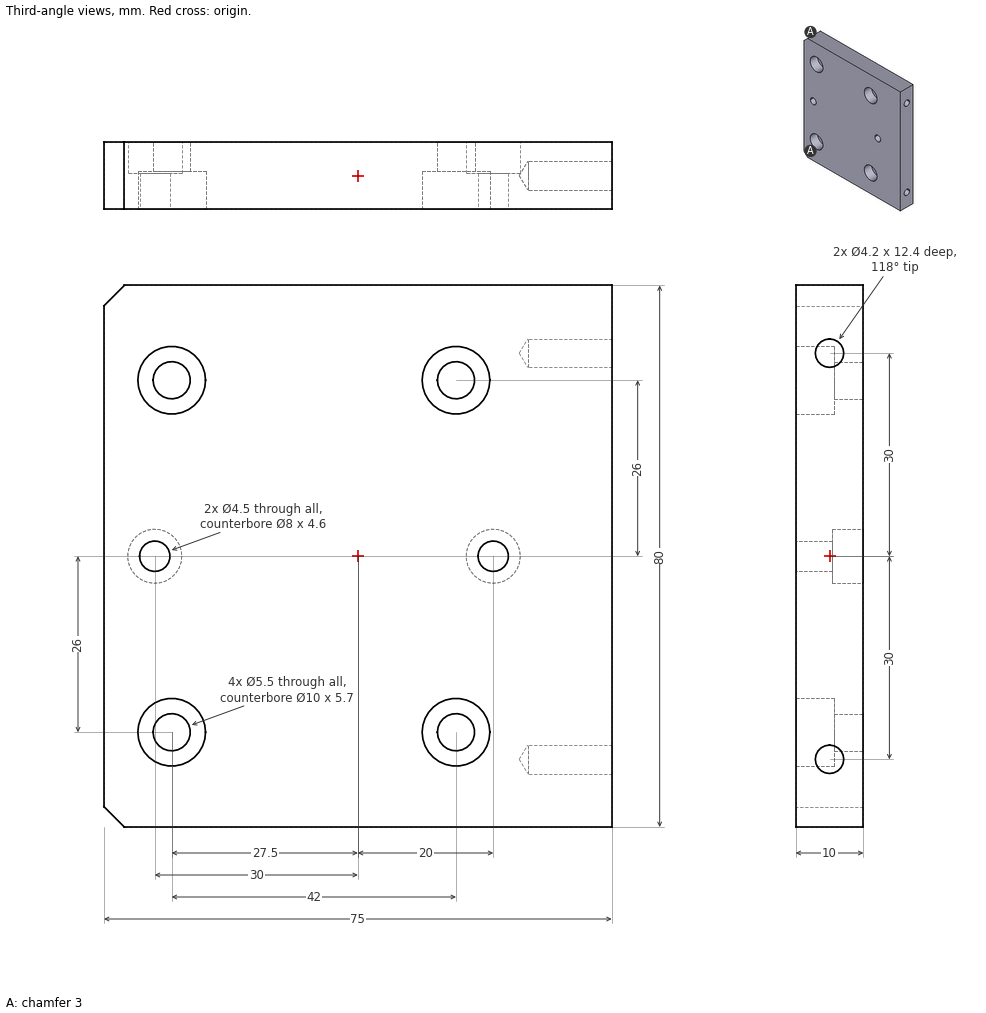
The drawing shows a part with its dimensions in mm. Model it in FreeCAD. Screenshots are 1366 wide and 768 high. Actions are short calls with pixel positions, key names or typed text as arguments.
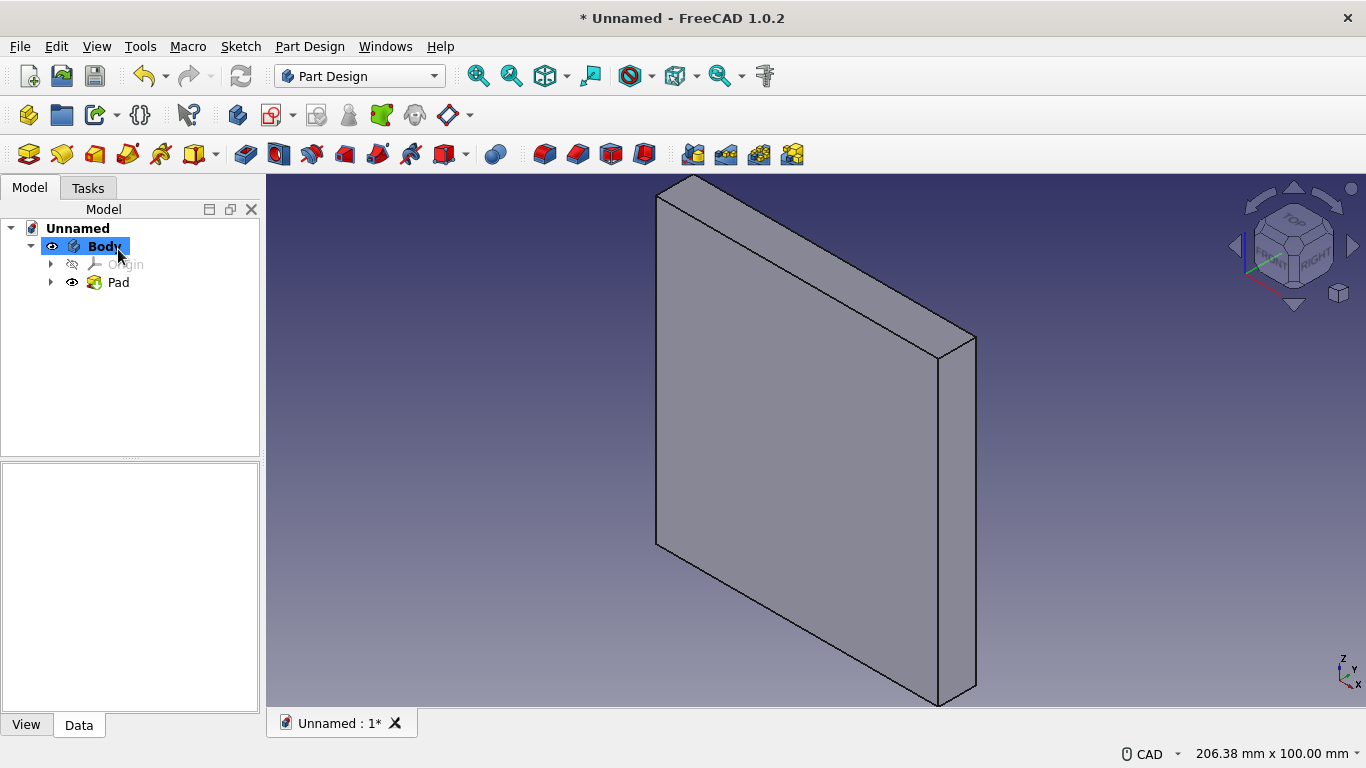
click(479, 76)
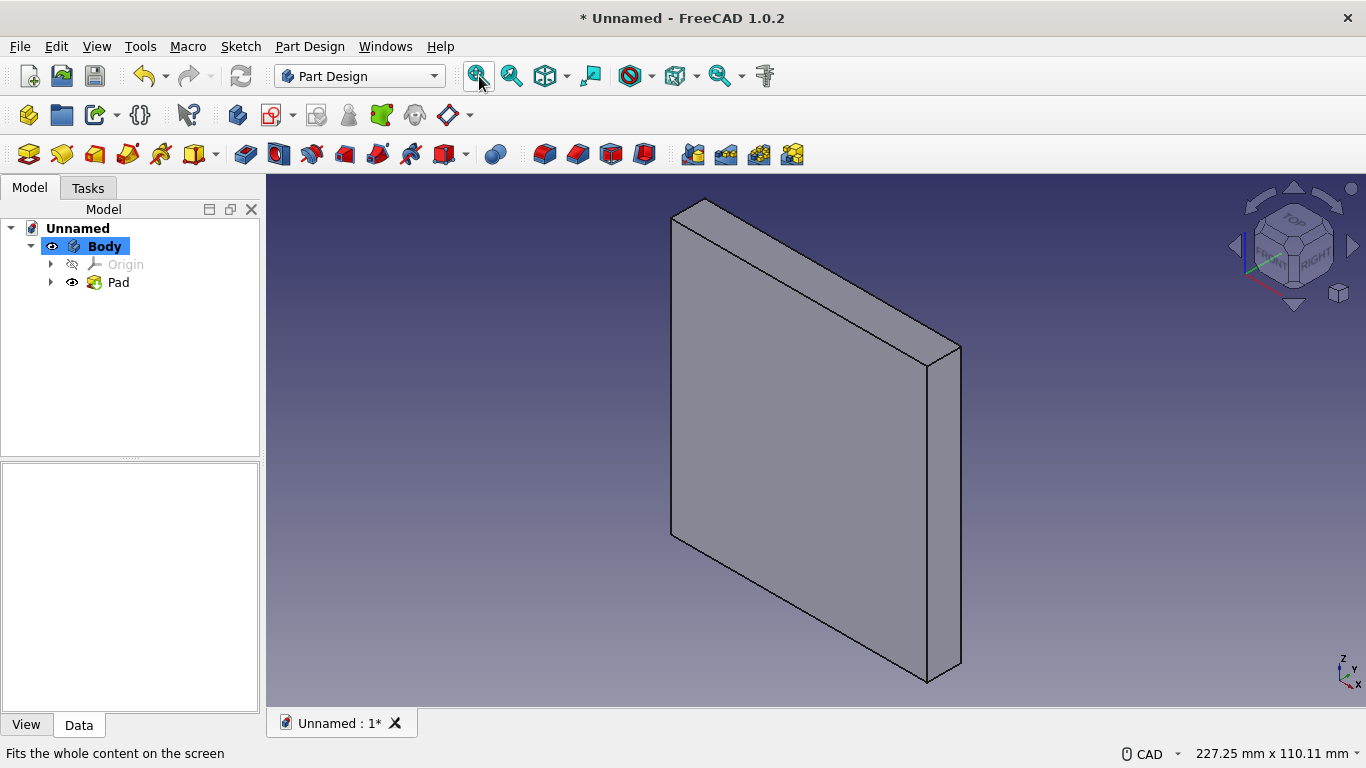
key(2)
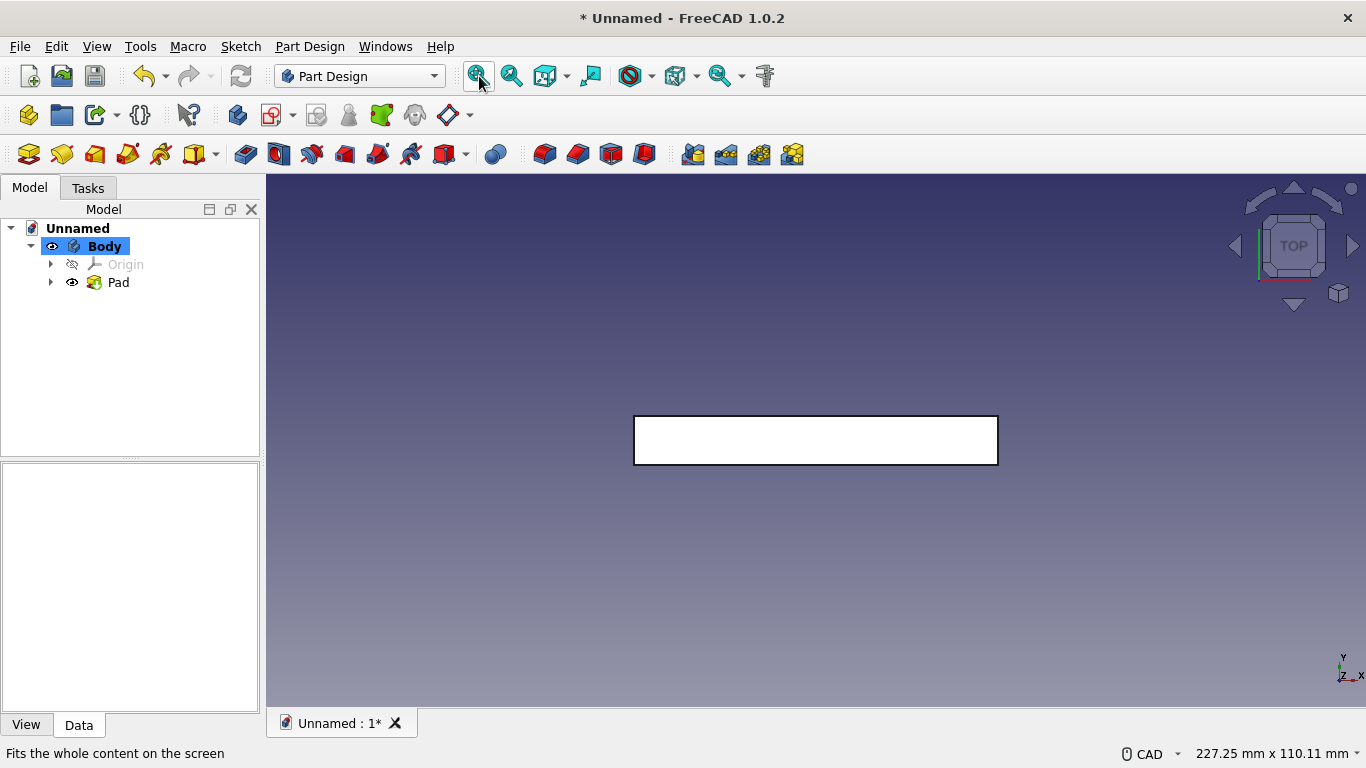
click(479, 76)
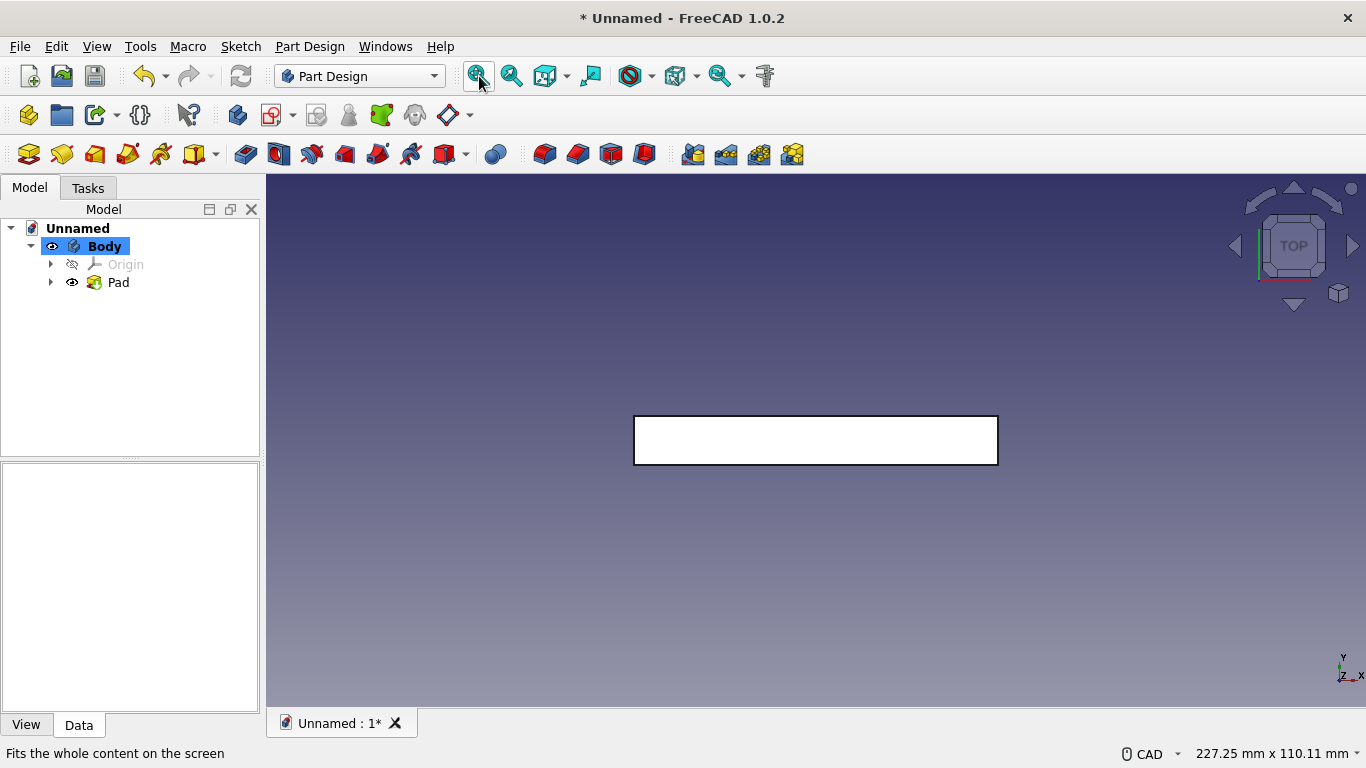
click(634, 439)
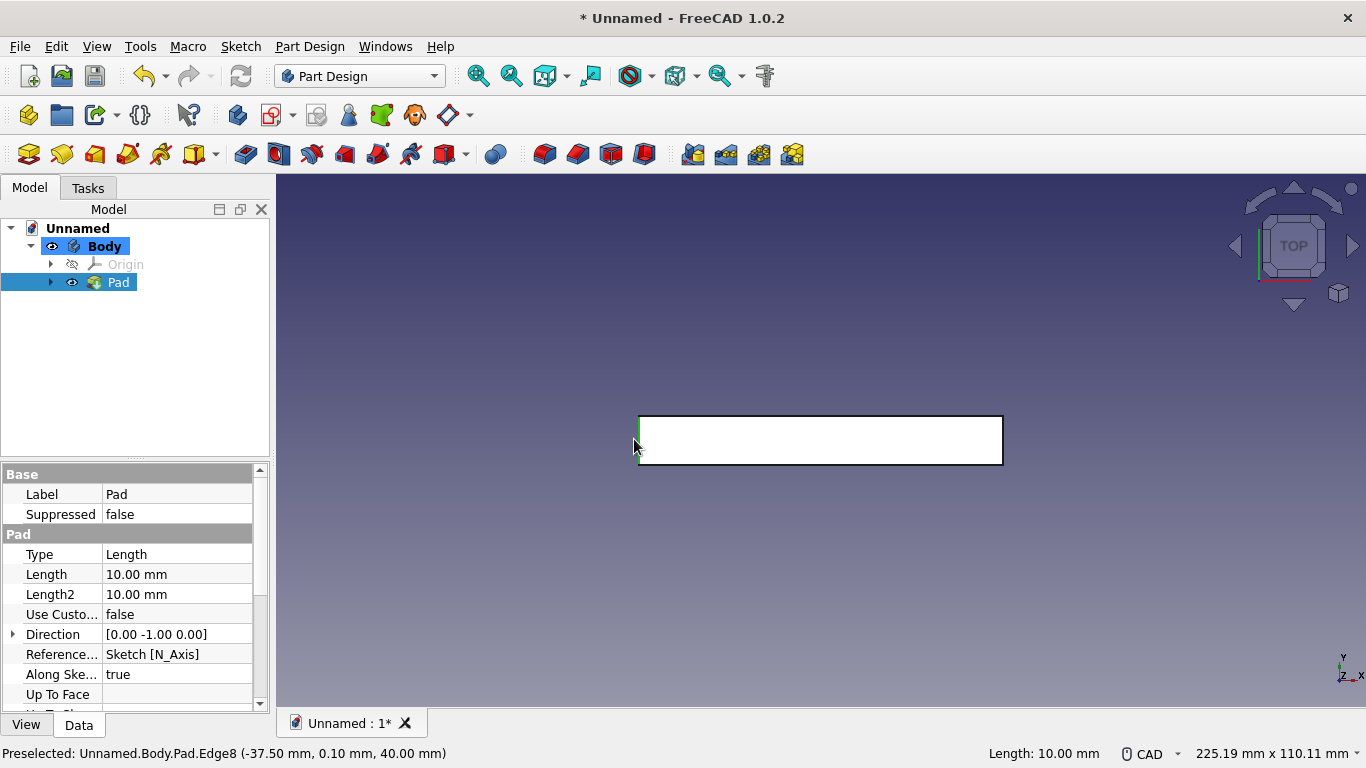
key(1)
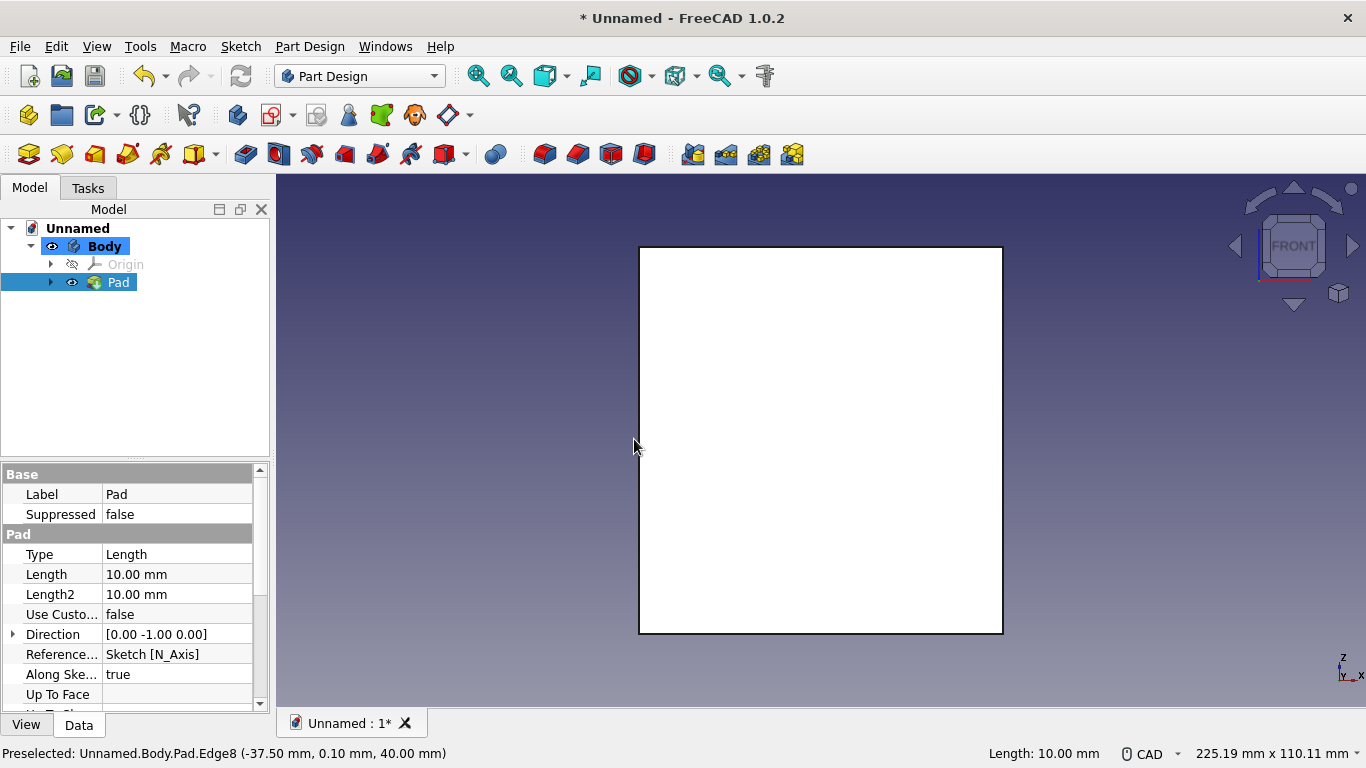
key(3)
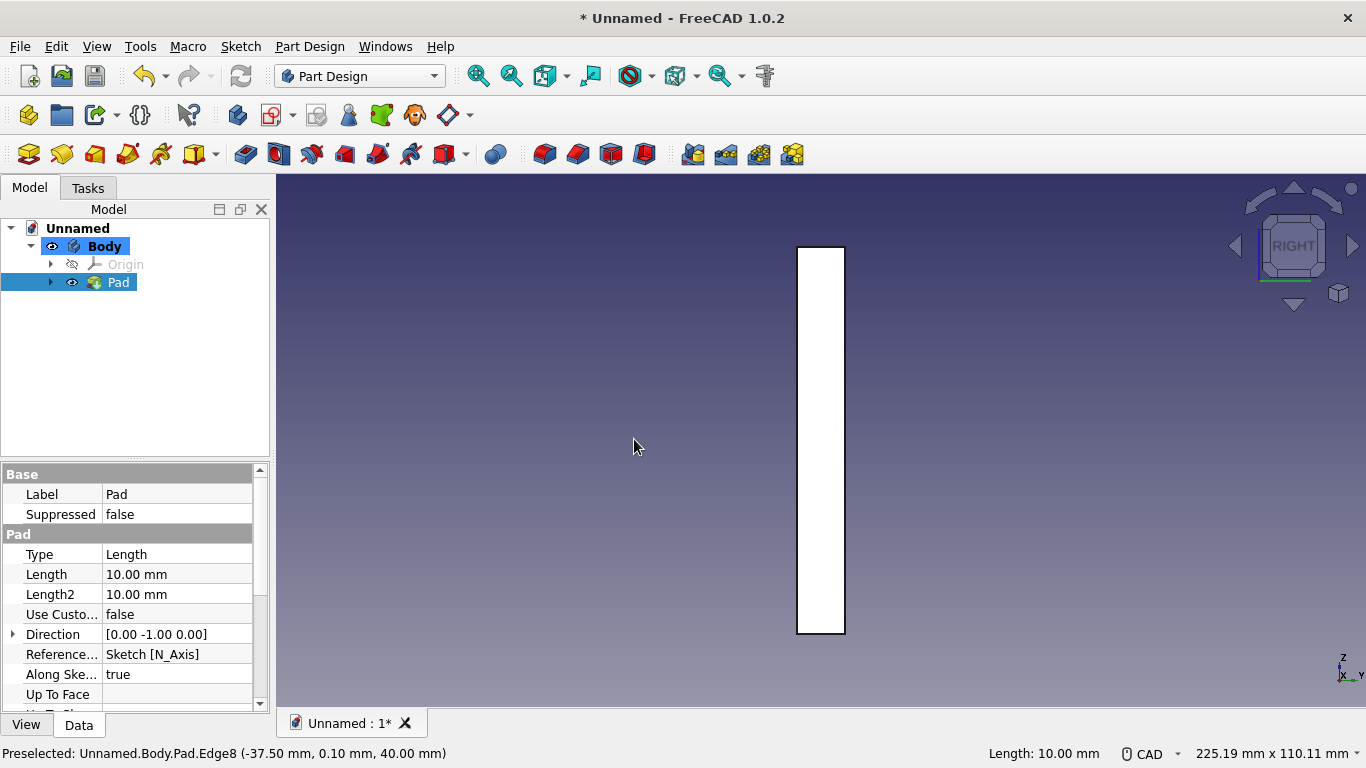
key(5)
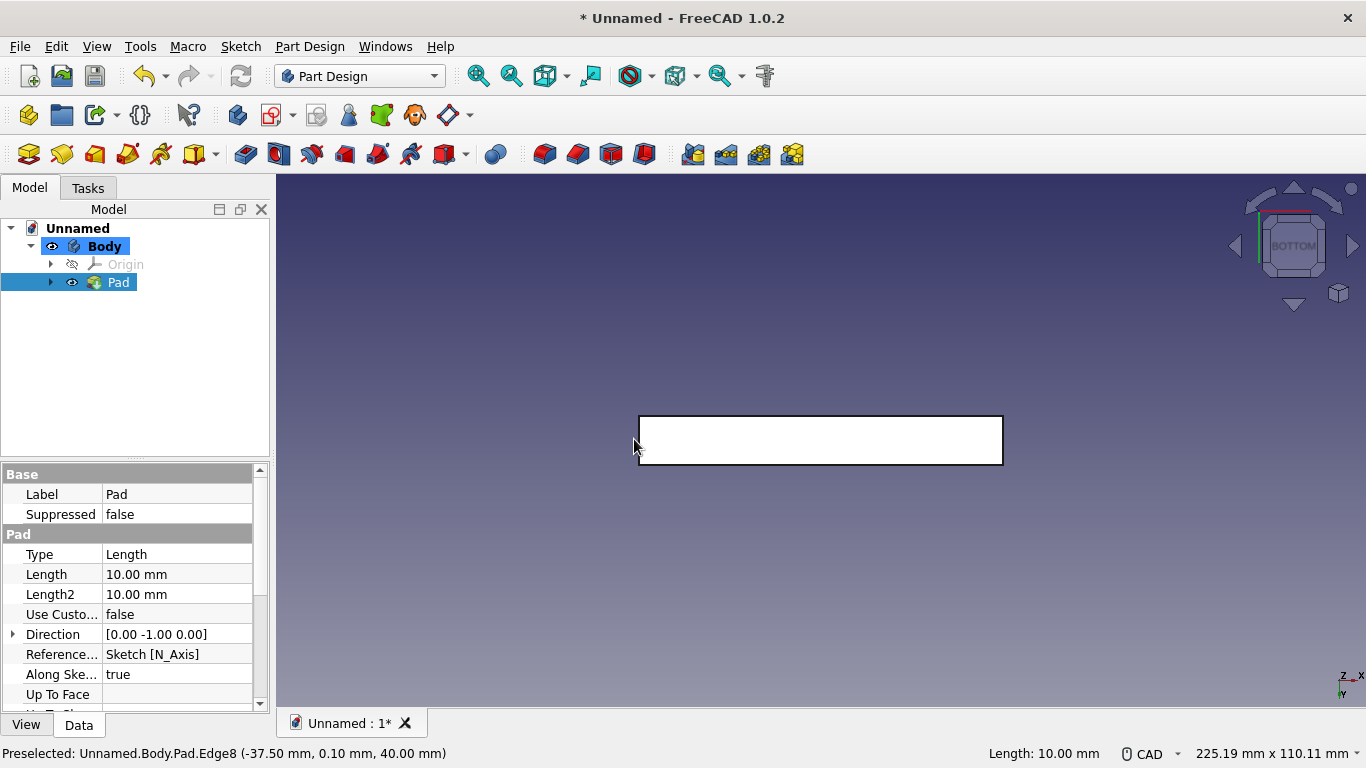
click(479, 76)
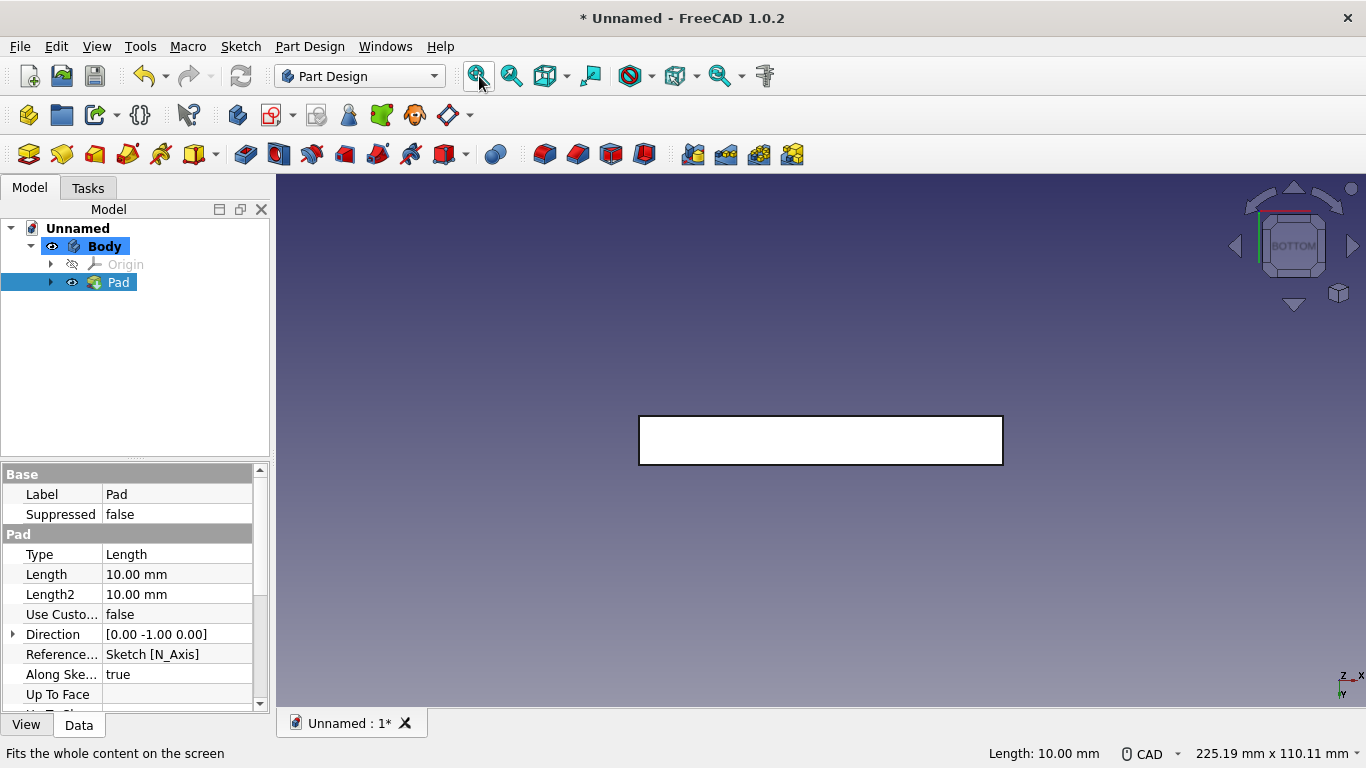
click(639, 439, ctrl)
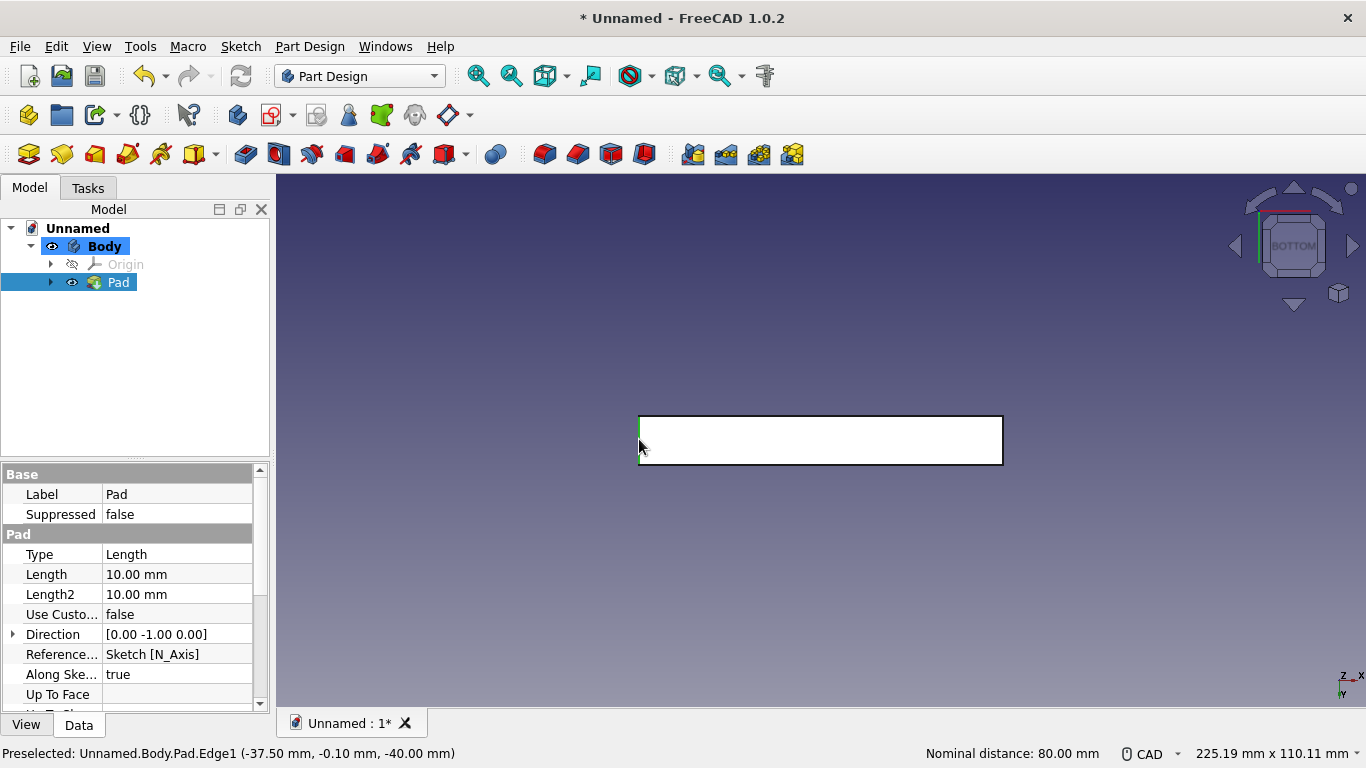
click(578, 154)